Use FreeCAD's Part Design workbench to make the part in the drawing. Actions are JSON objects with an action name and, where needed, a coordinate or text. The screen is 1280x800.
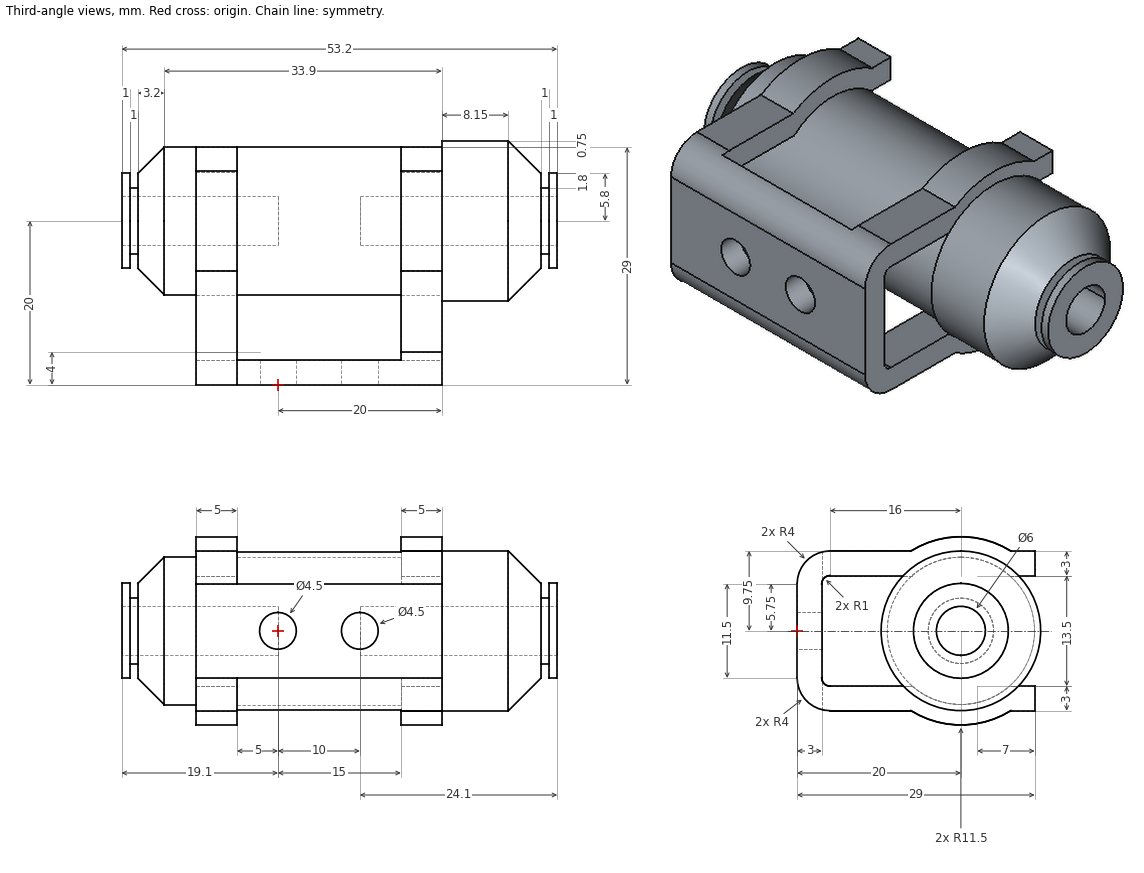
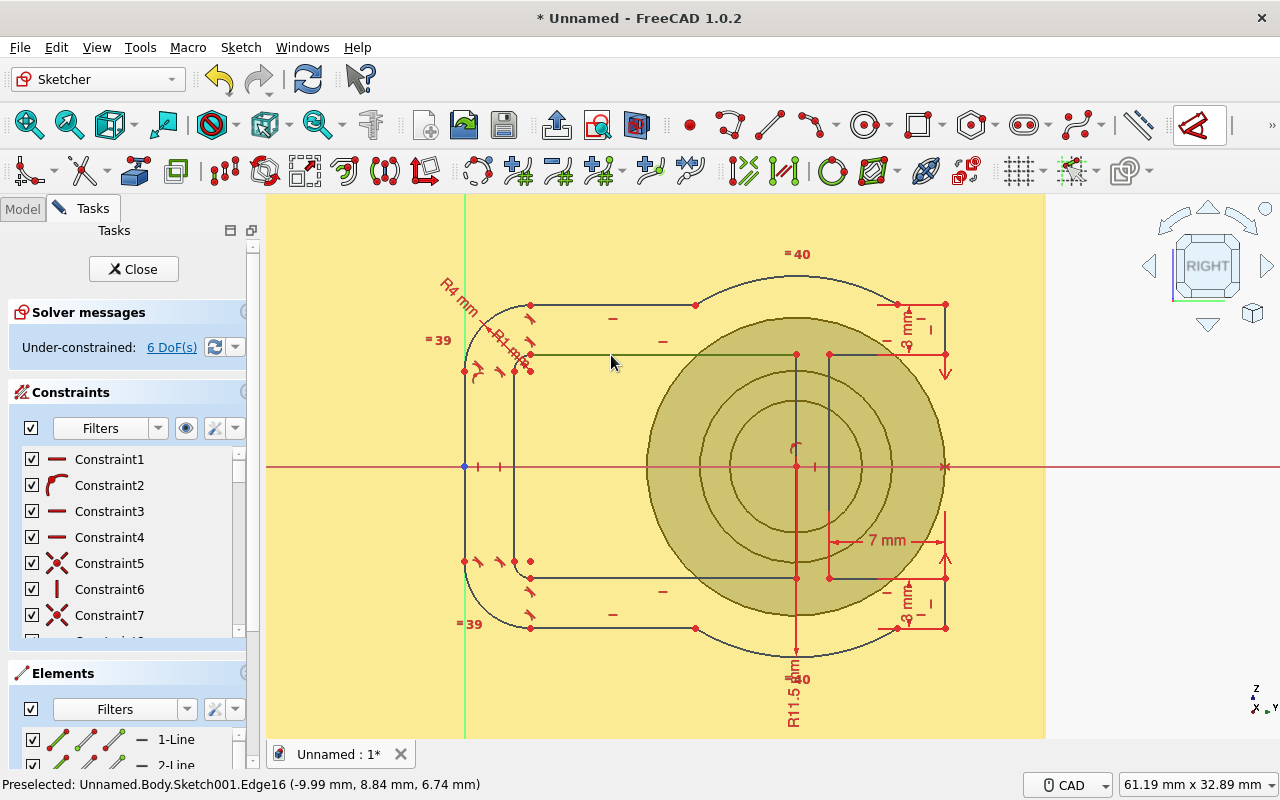
{"action": "key", "text": "l"}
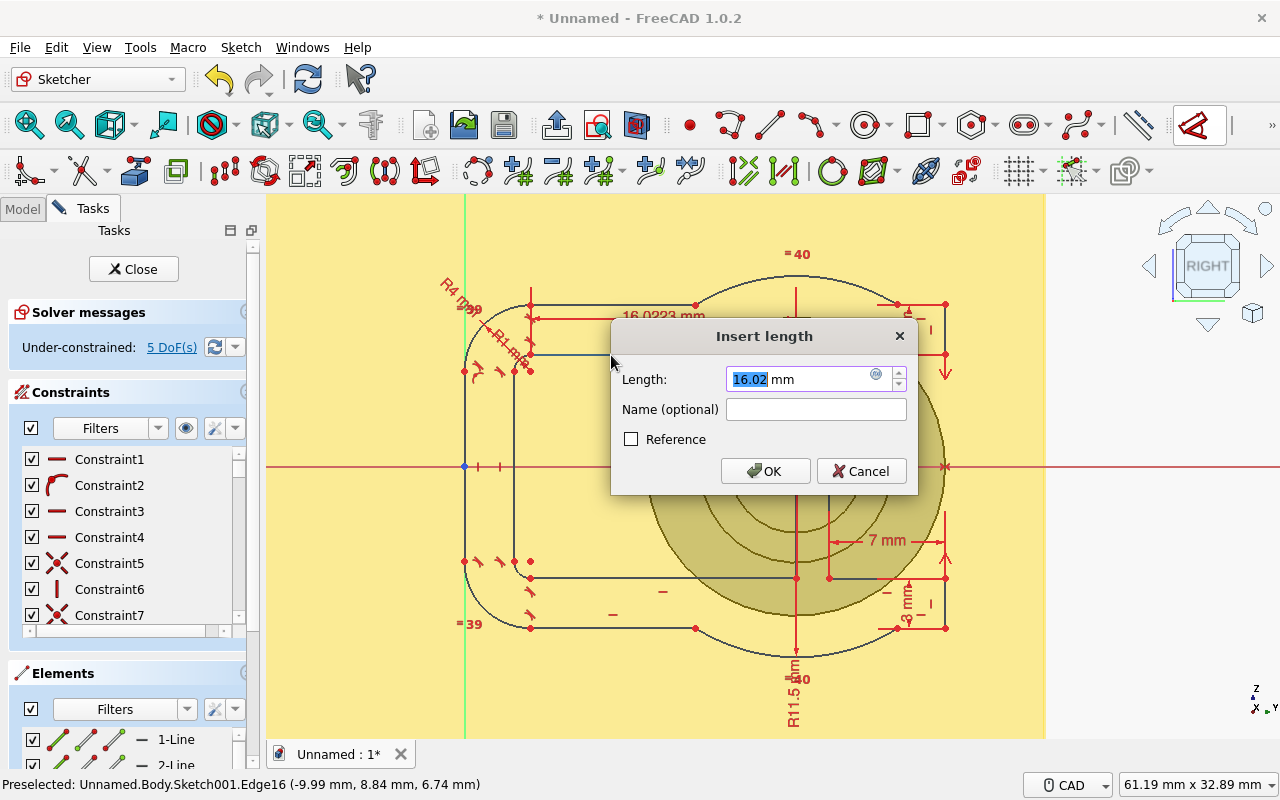
{"action": "type", "text": "16"}
{"action": "key", "text": "Return"}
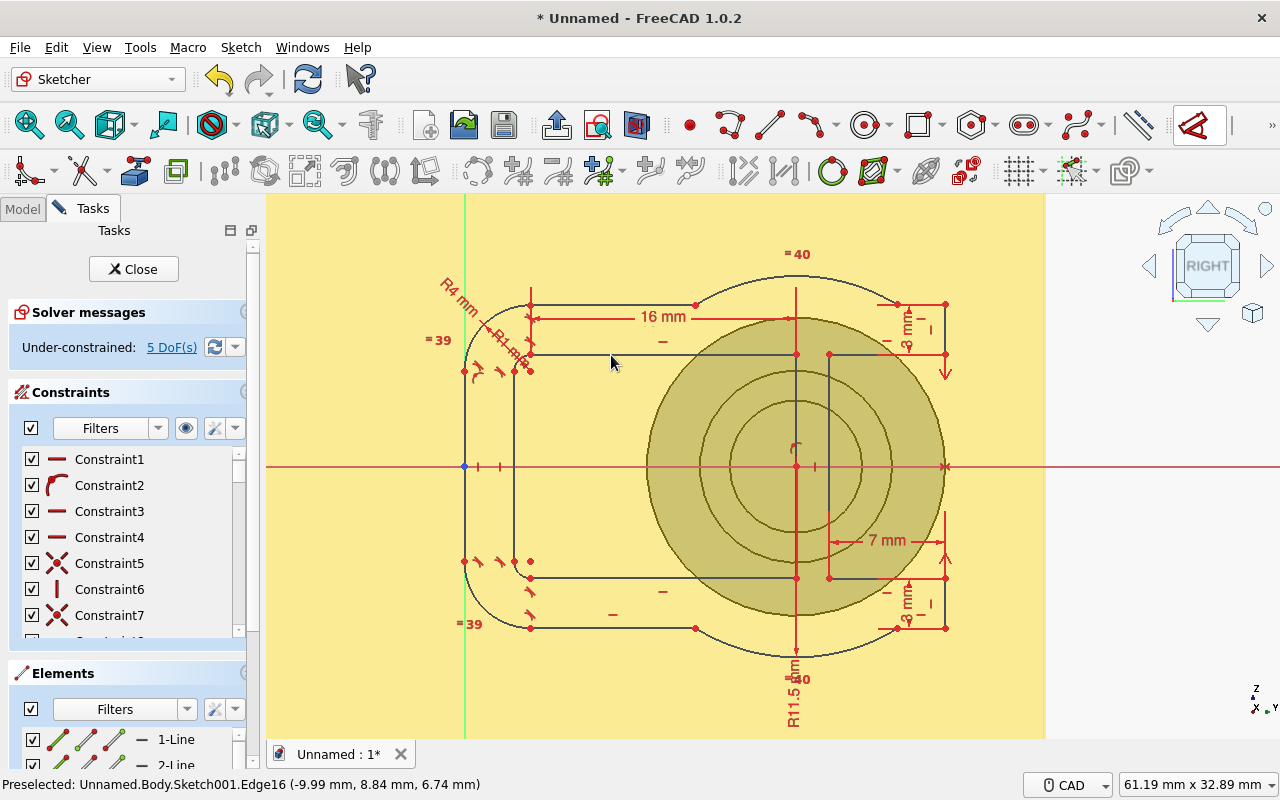
{"action": "left_click", "coordinate": [945, 628]}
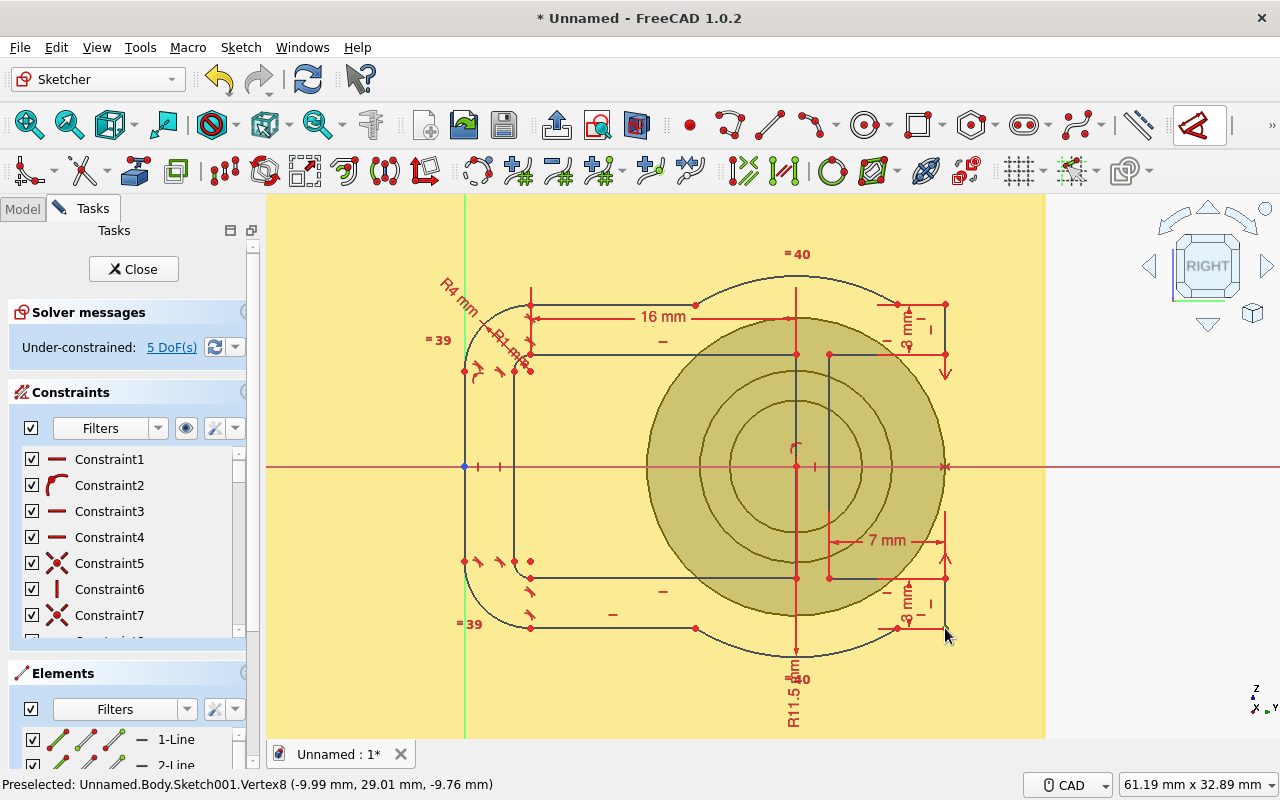
{"action": "left_click", "coordinate": [1220, 126]}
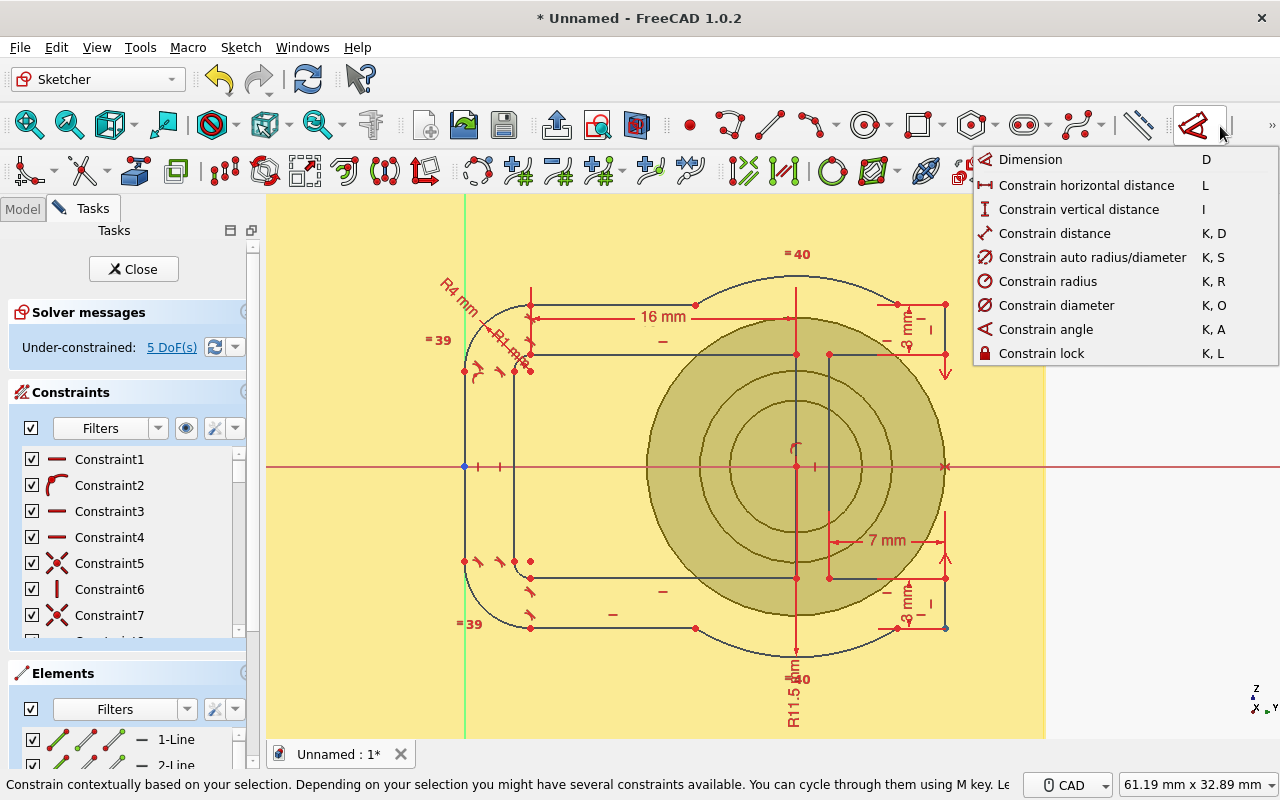
{"action": "left_click", "coordinate": [1126, 185]}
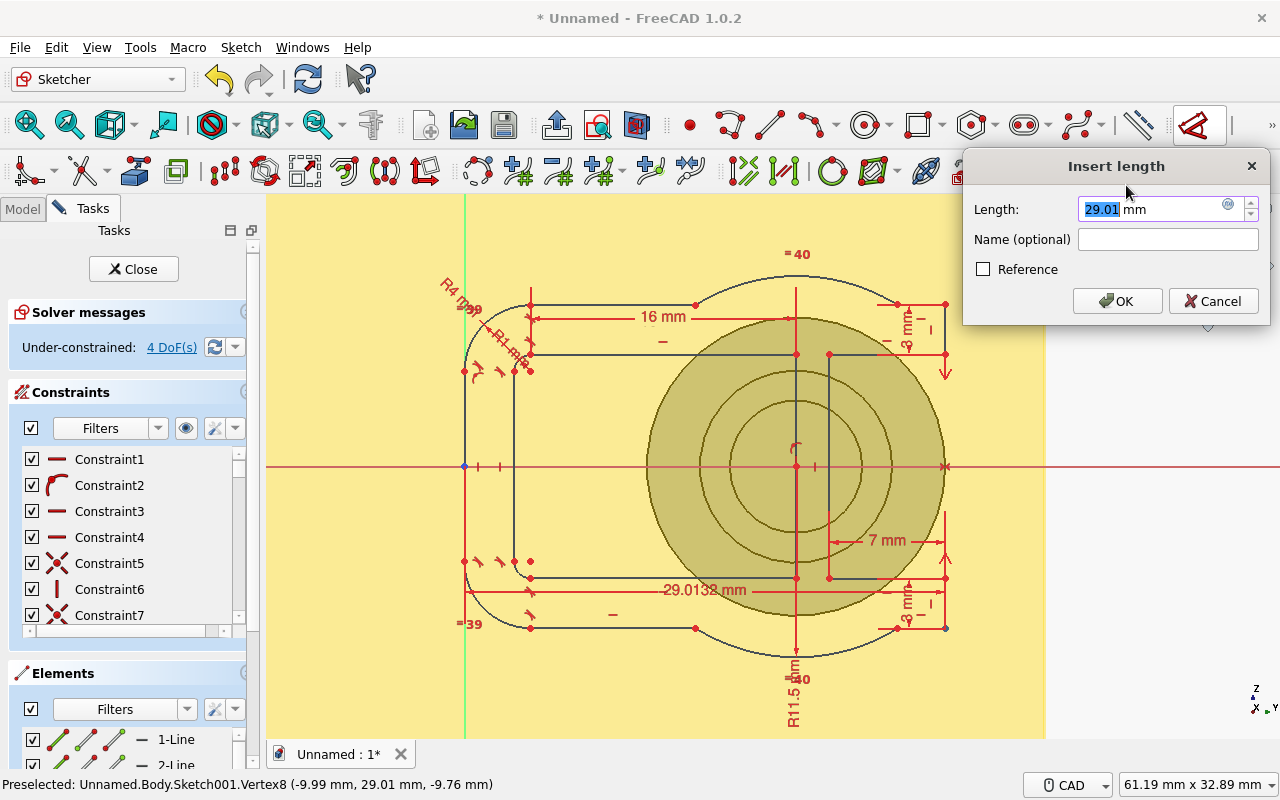
{"action": "type", "text": "29"}
{"action": "key", "text": "Return"}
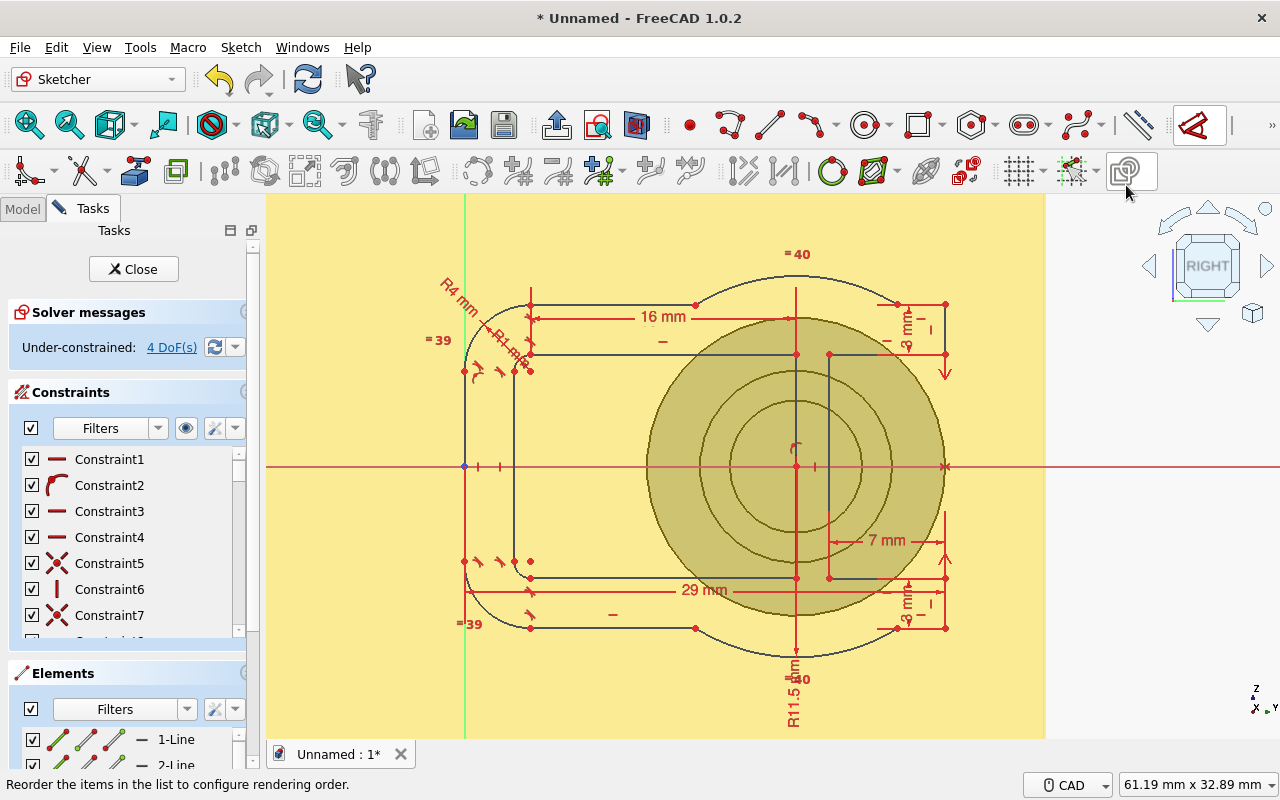
{"action": "left_click", "coordinate": [797, 467]}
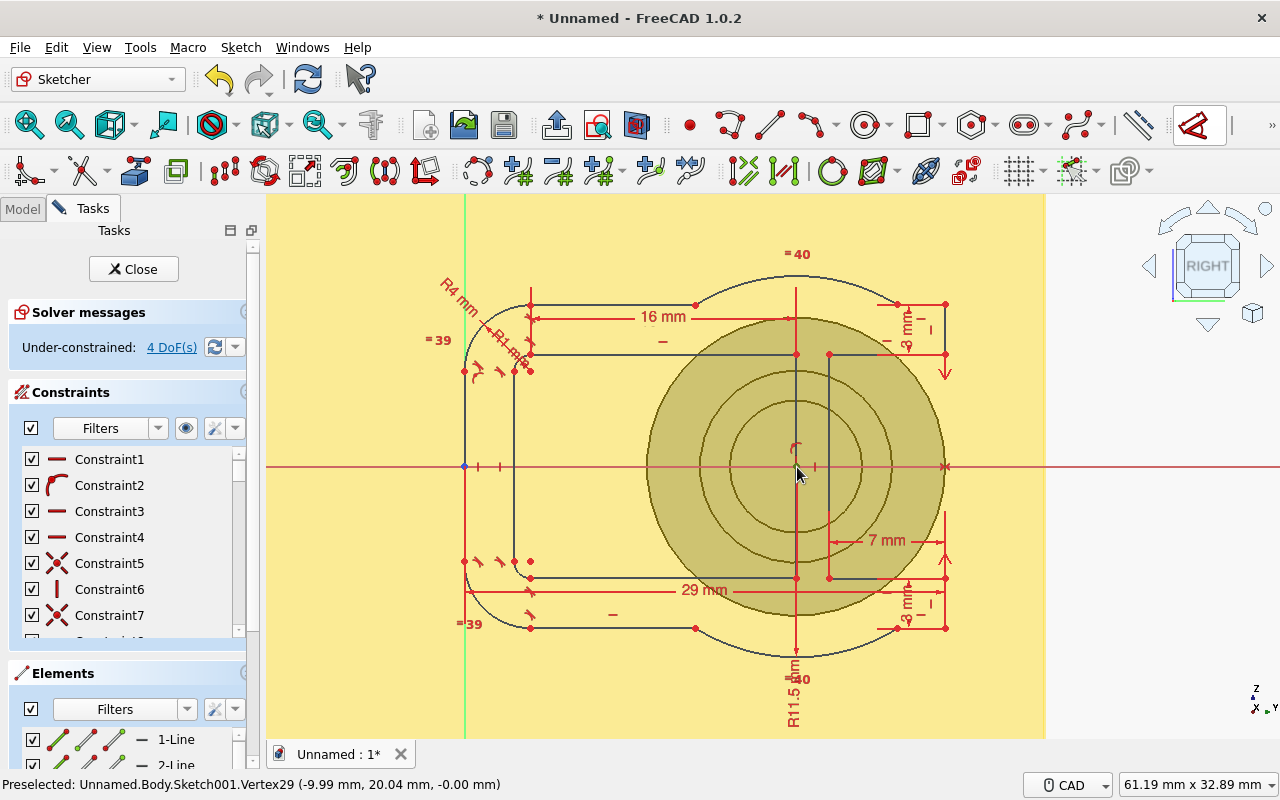
{"action": "key", "text": "l"}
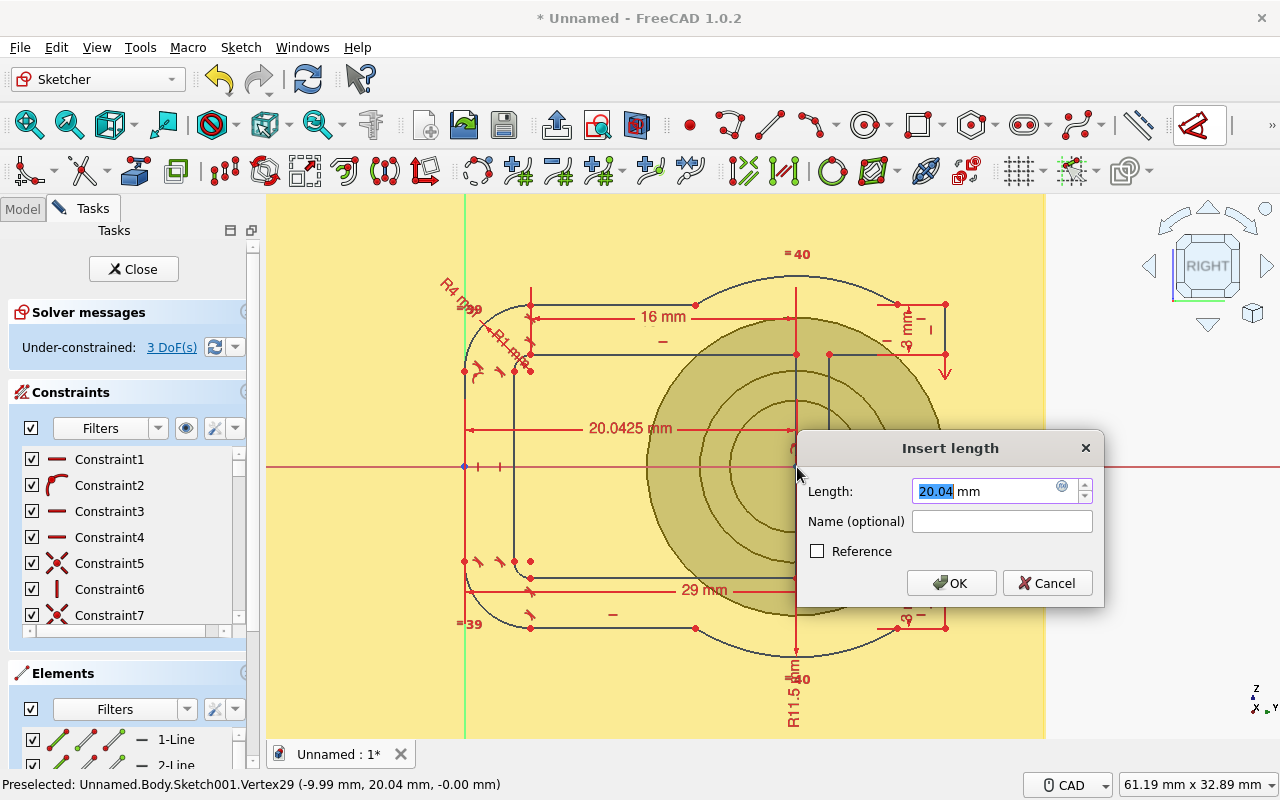
{"action": "type", "text": "20"}
{"action": "key", "text": "Return"}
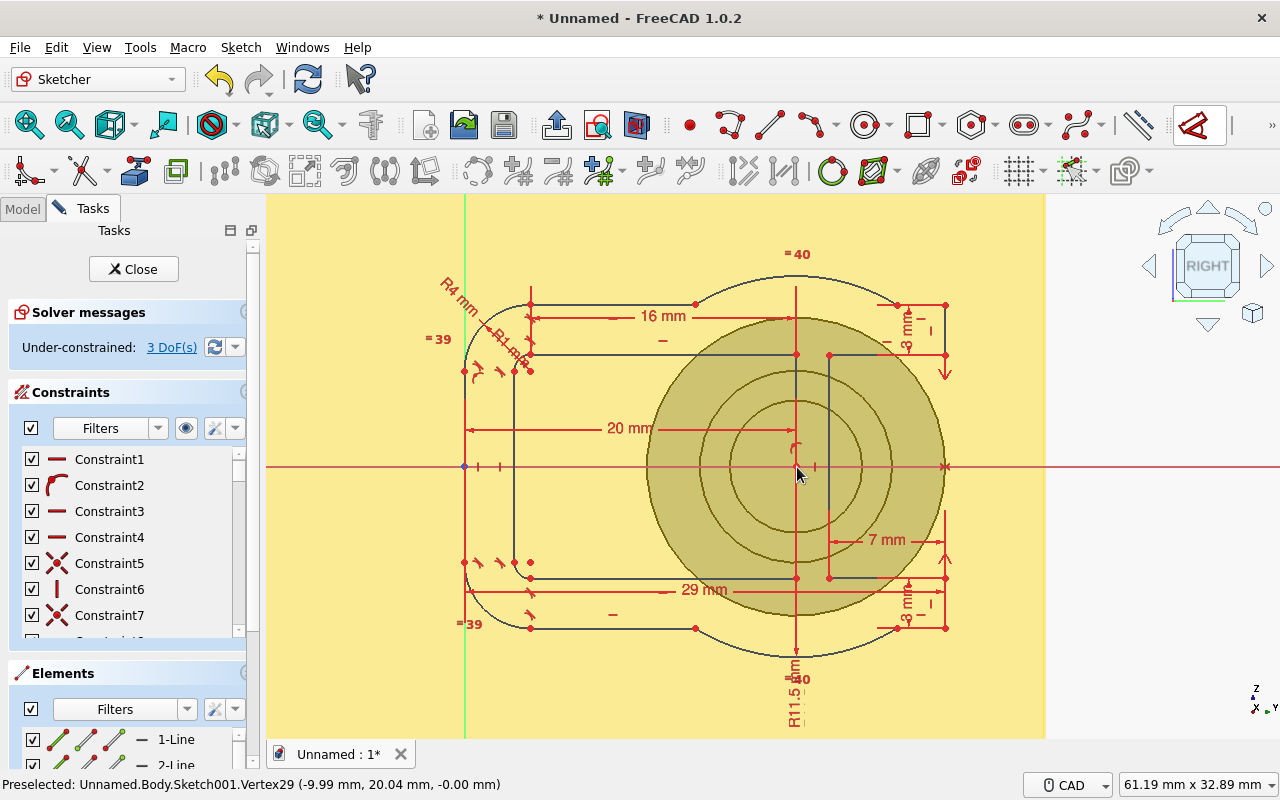
{"action": "left_click", "coordinate": [465, 428]}